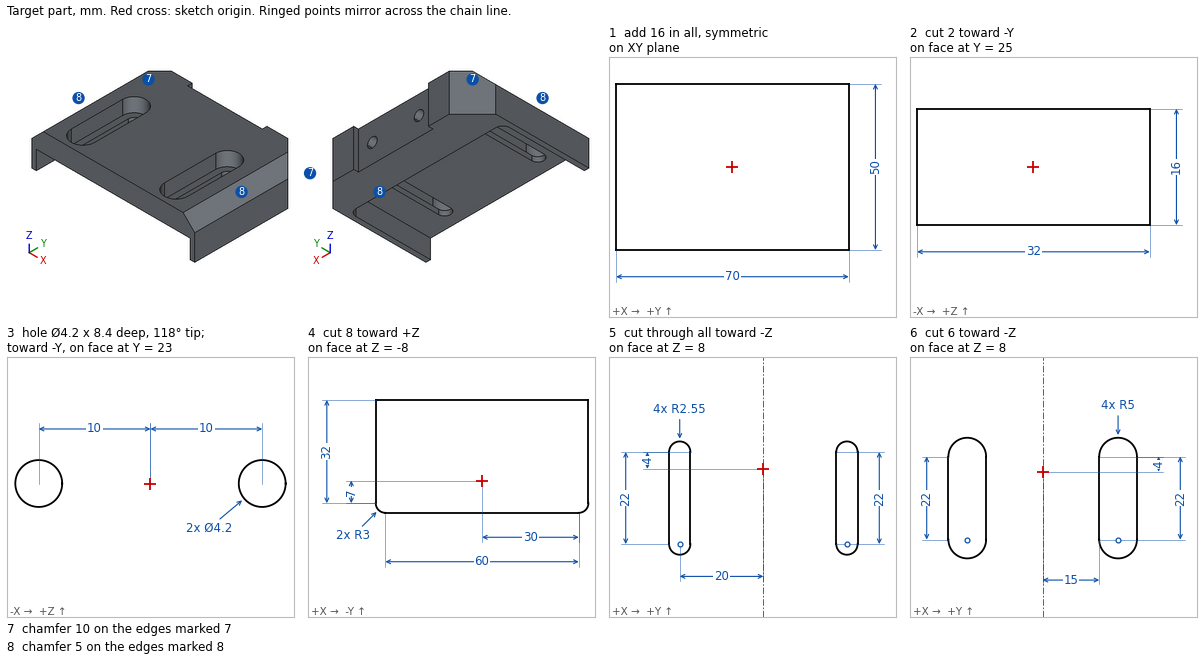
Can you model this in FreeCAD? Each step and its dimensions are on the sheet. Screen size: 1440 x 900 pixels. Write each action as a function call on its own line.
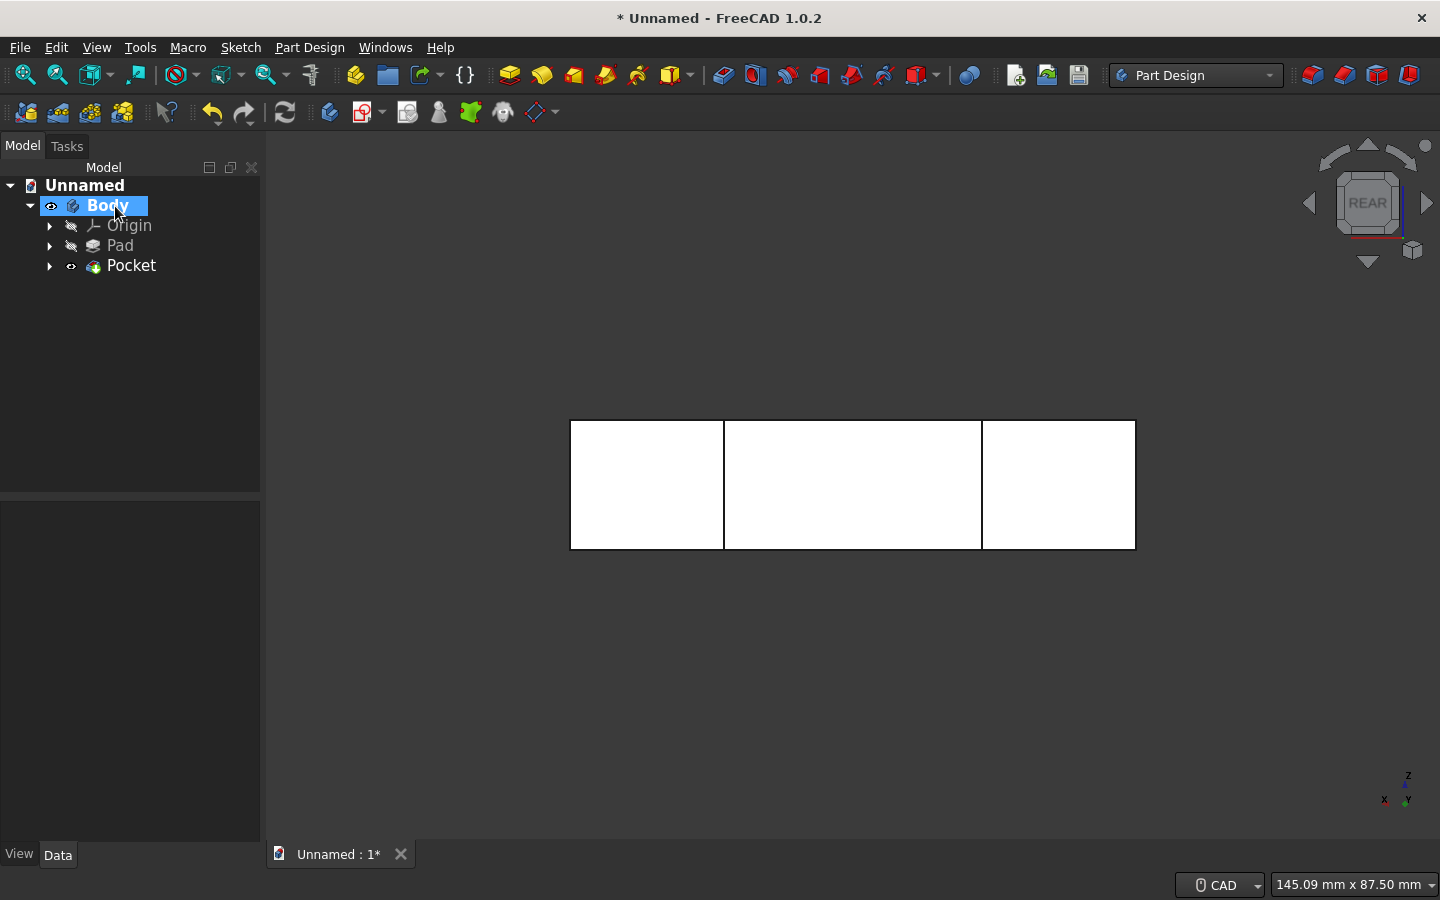
click(816, 484)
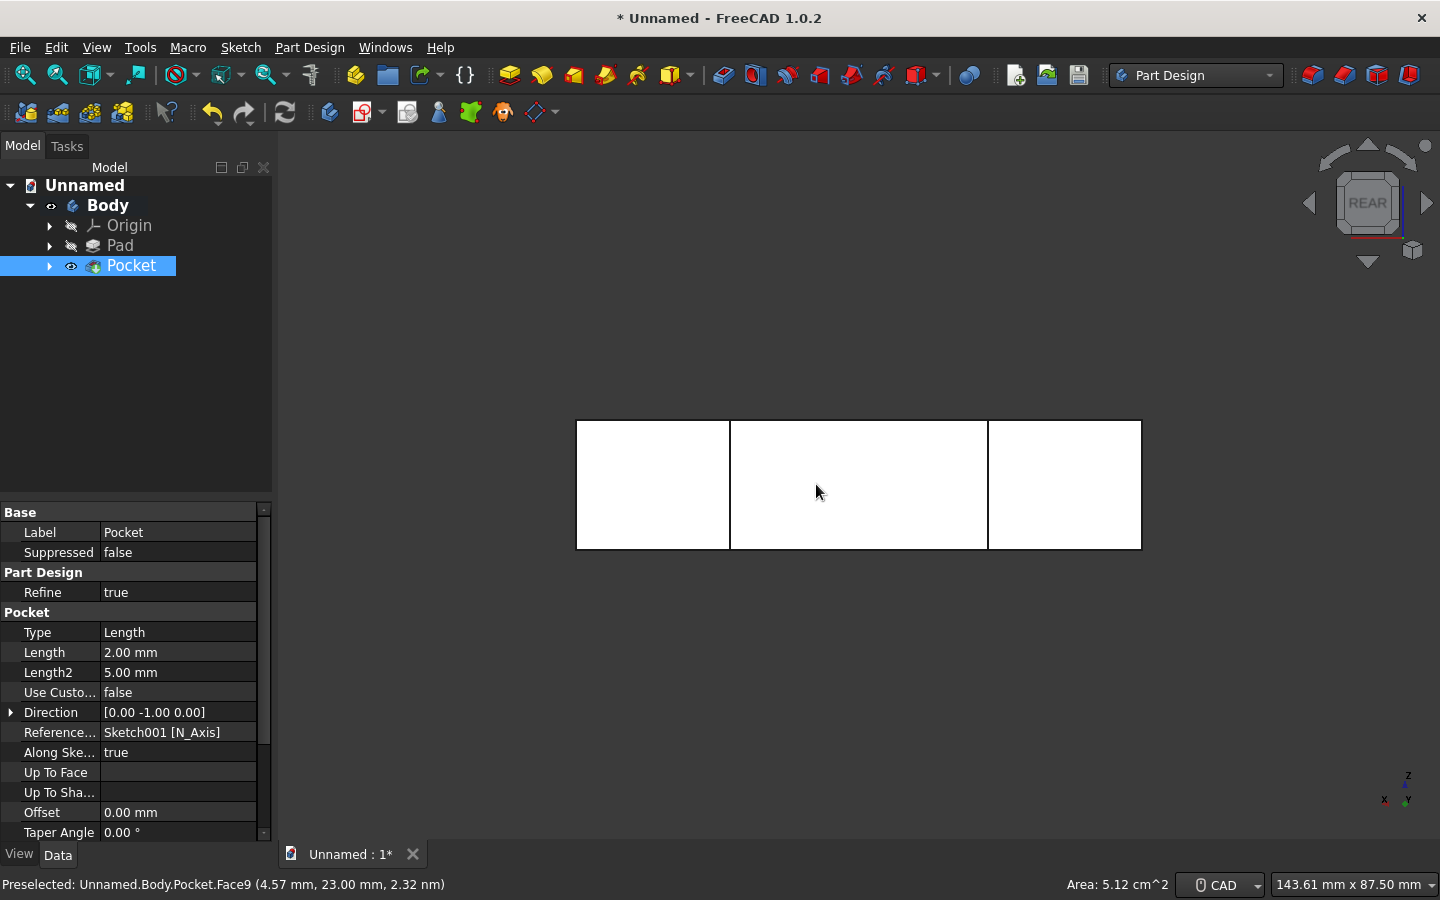
click(362, 112)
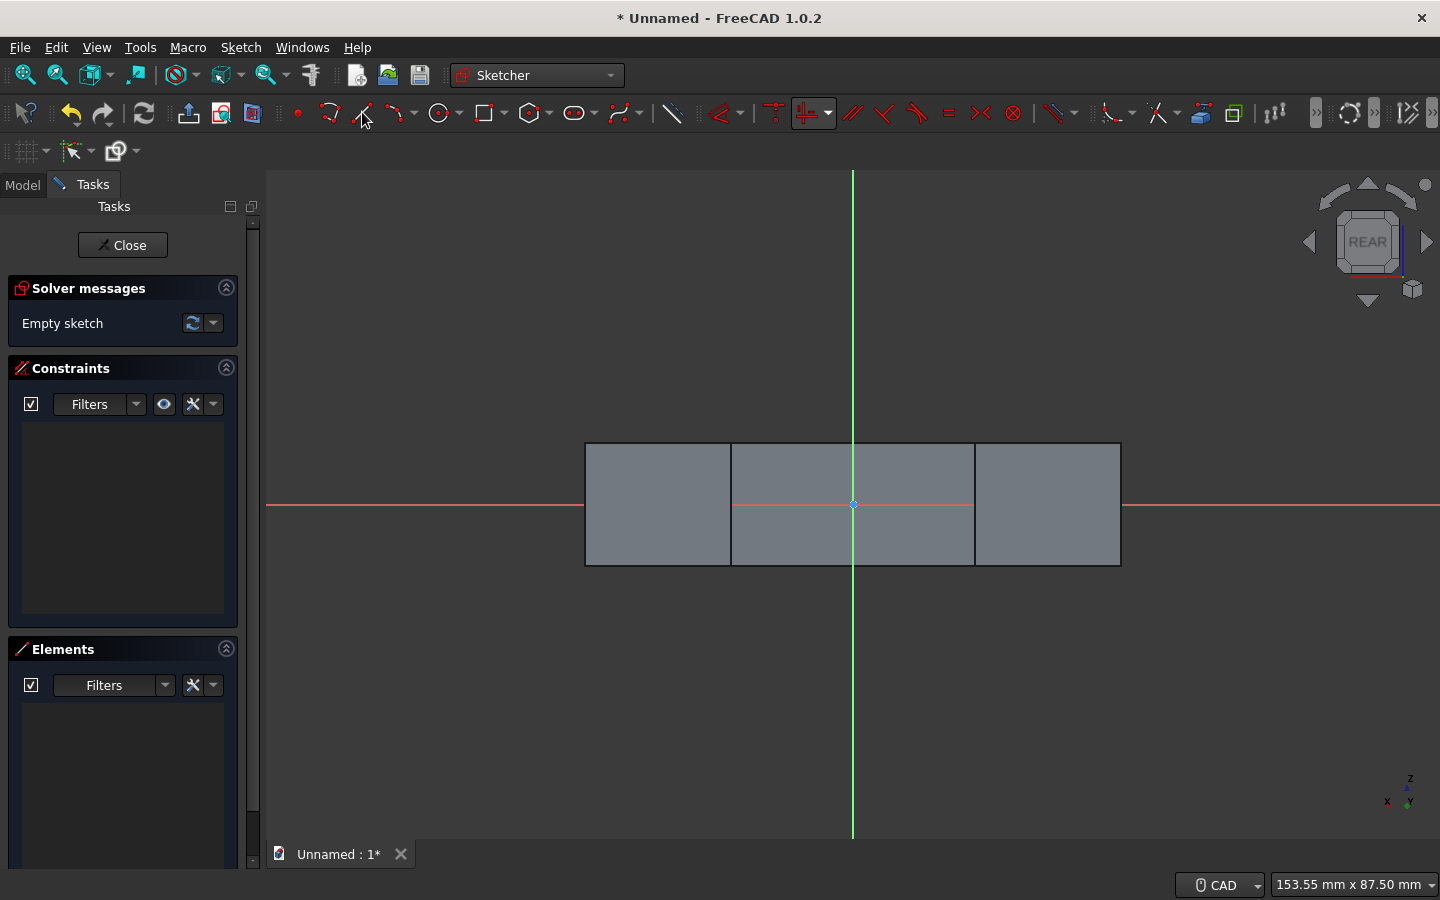
click(254, 114)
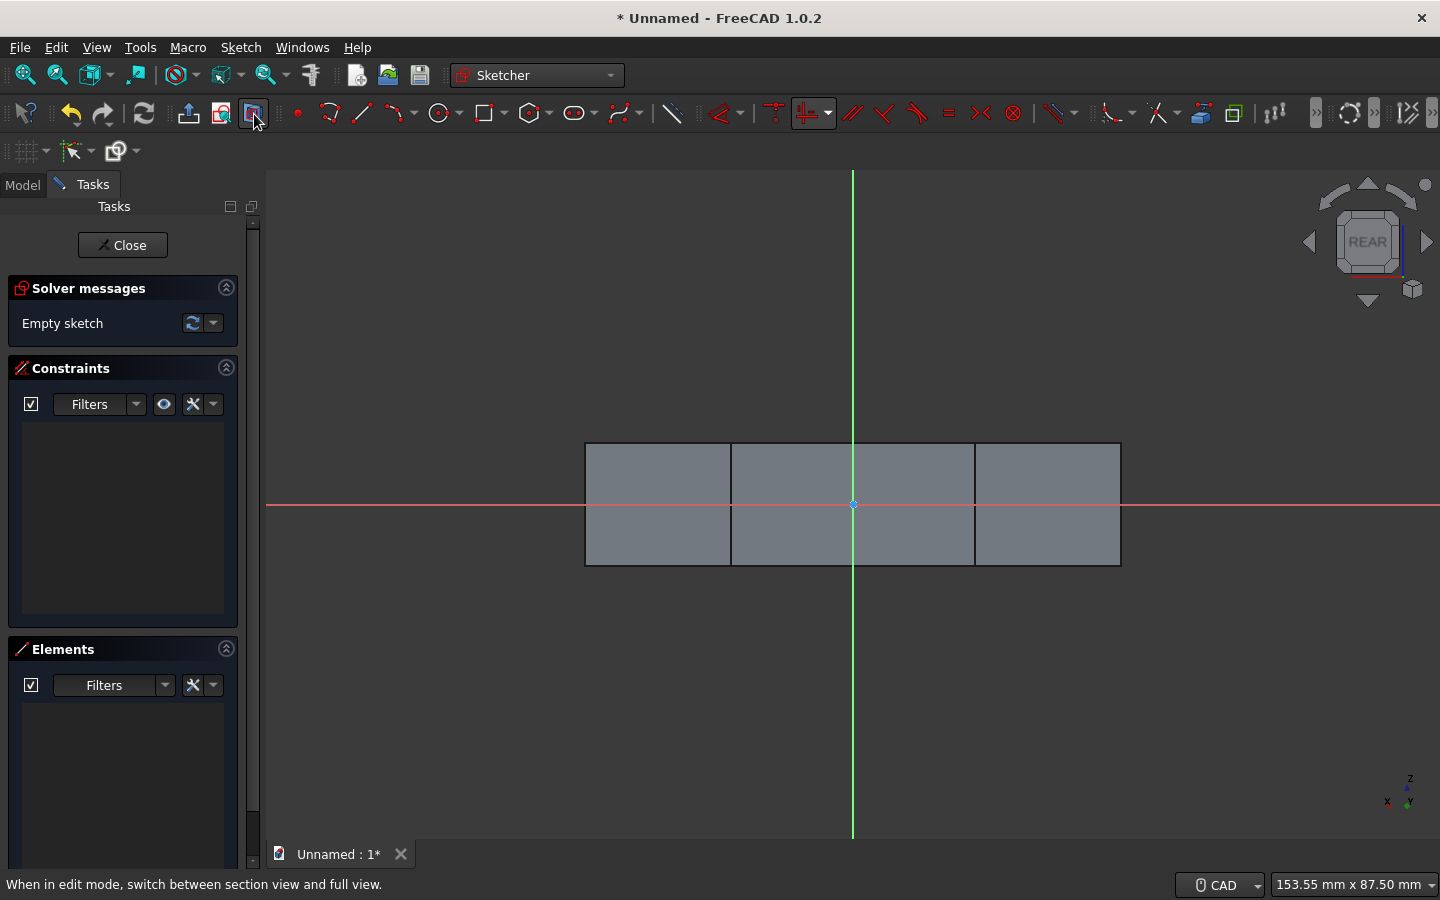
scroll(875, 505, up, 7)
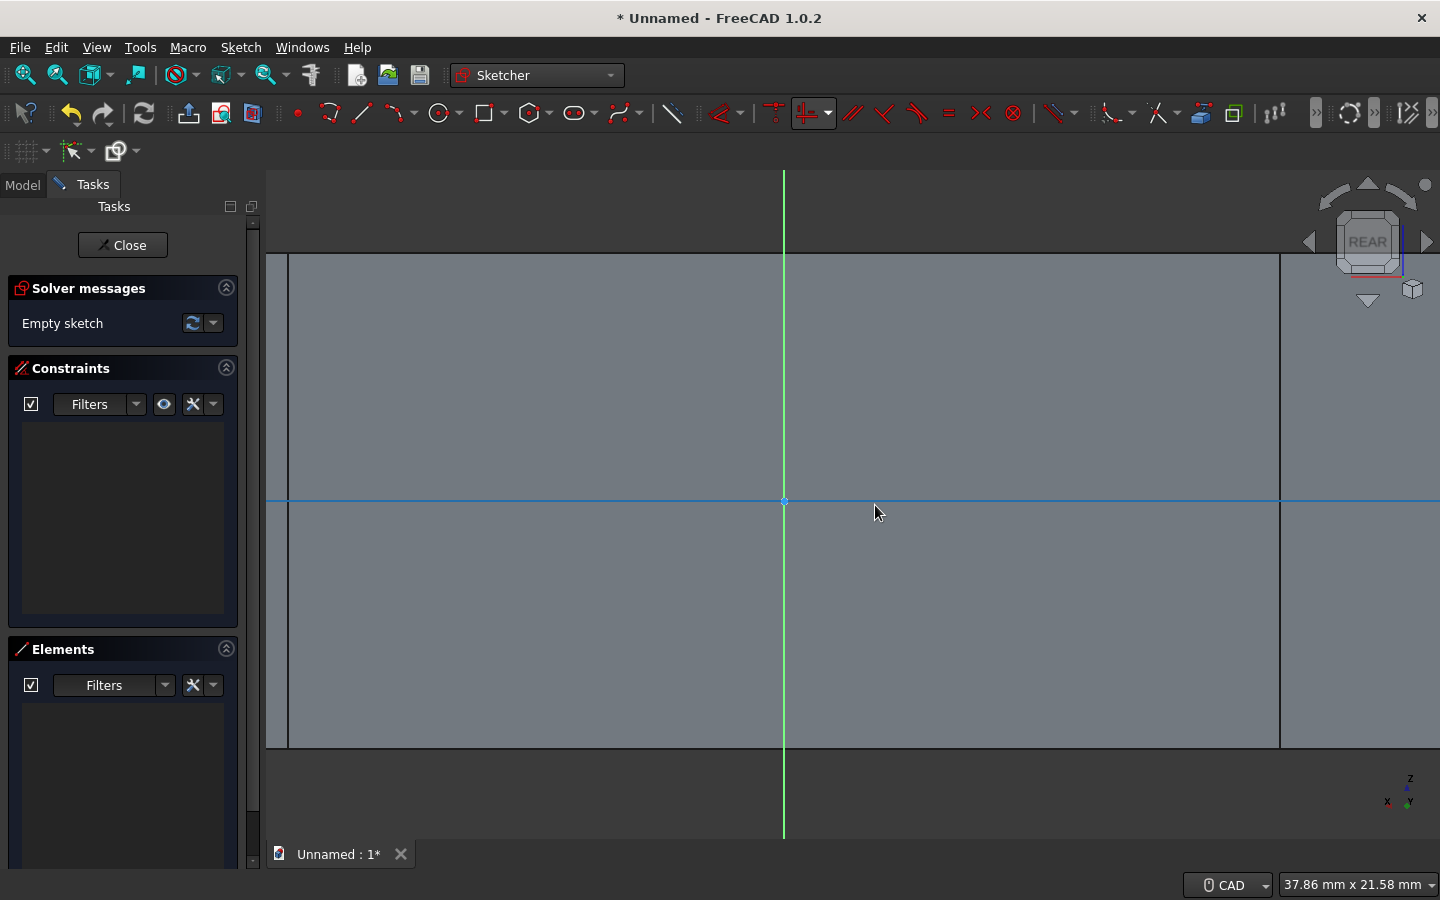
key(g)
key(c)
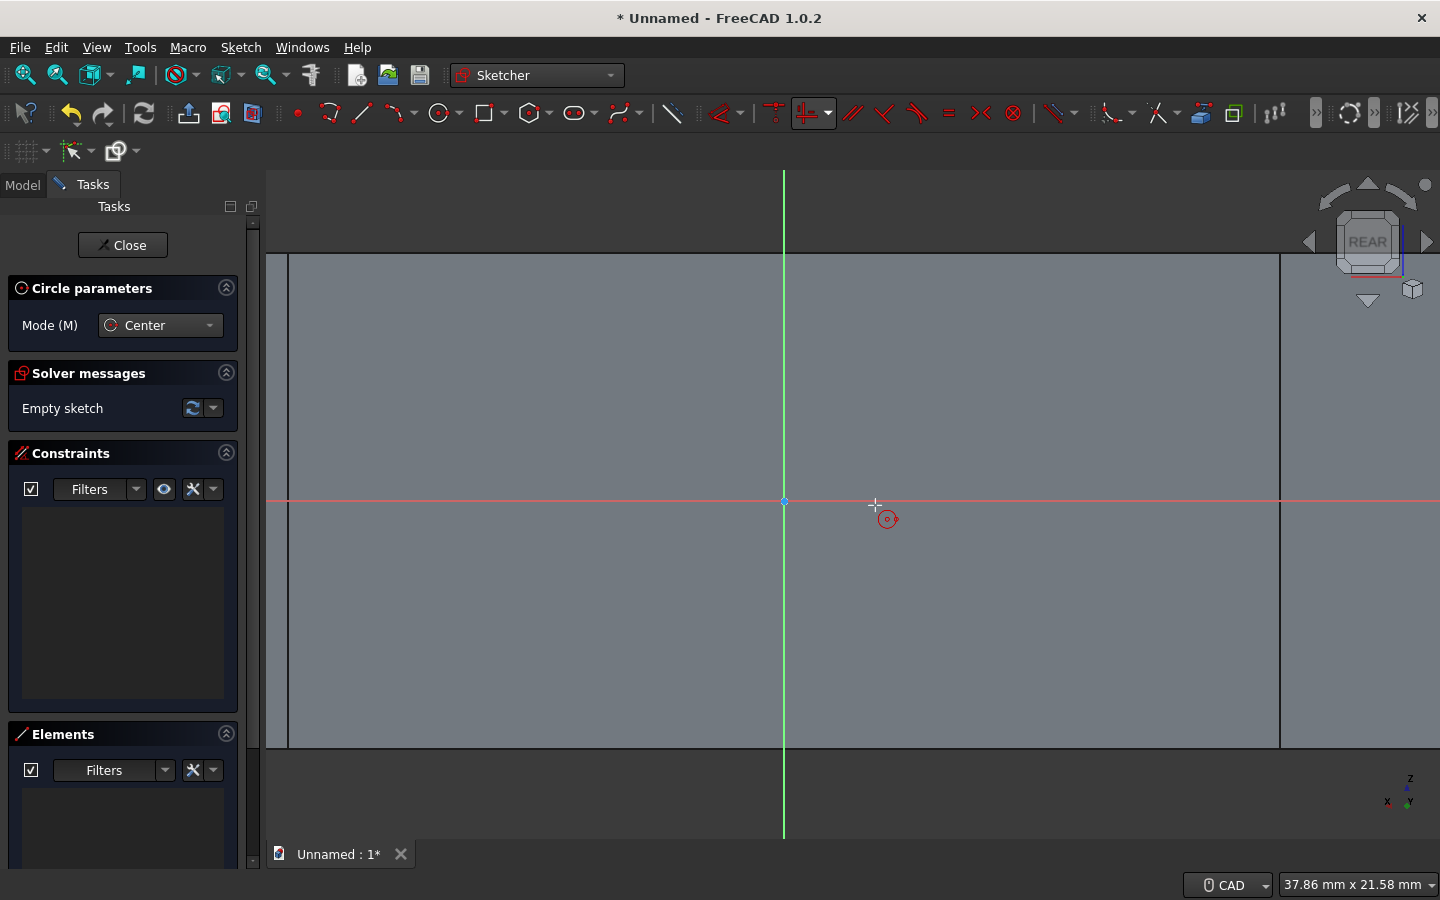
click(1094, 501)
move(1140, 455)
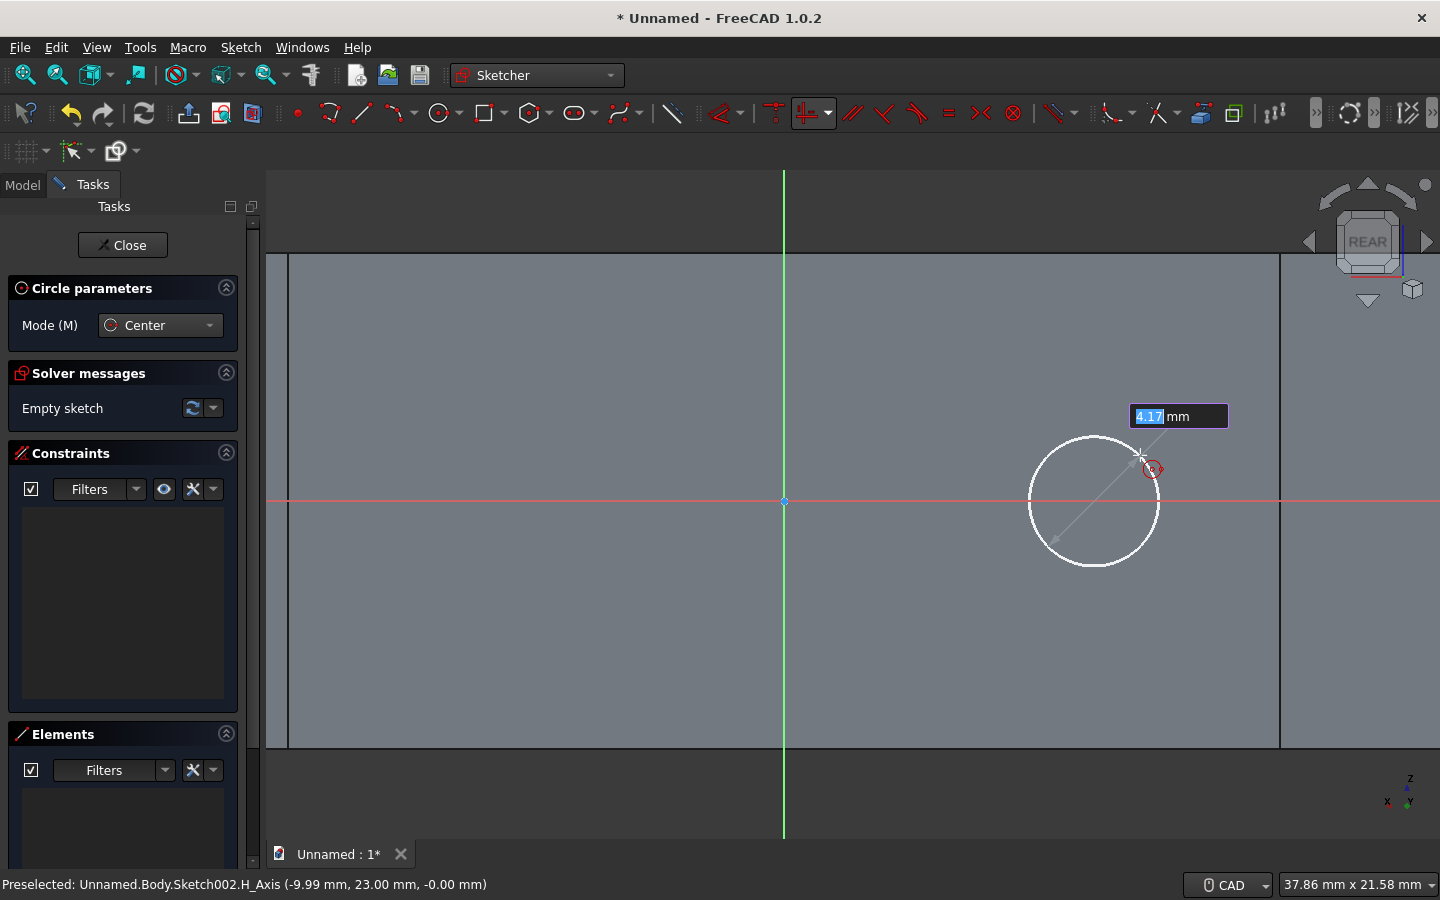
text(4.2)
key(Return)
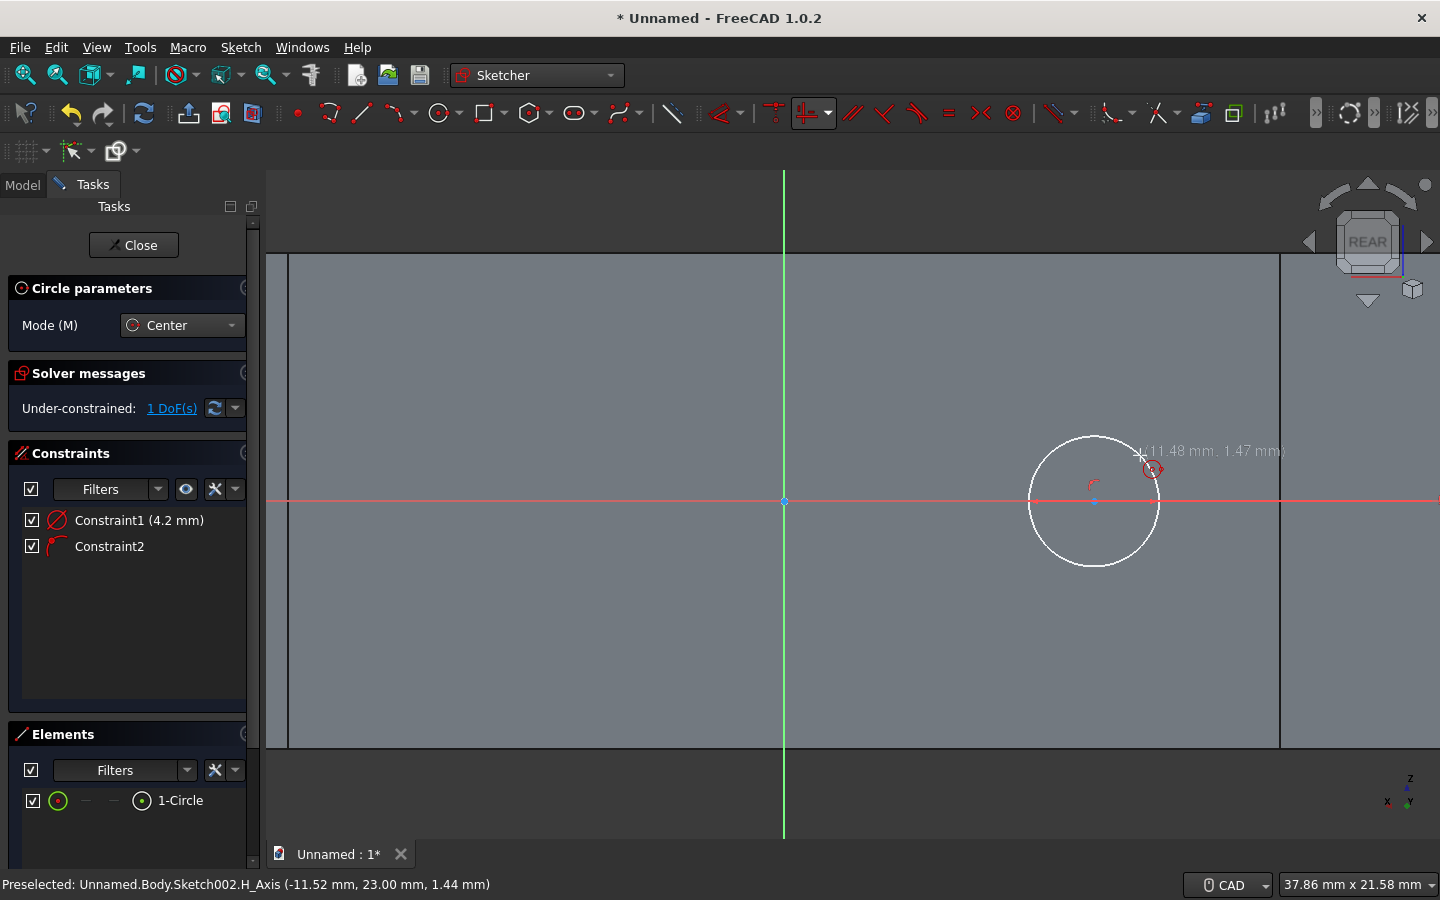
click(474, 501)
move(520, 455)